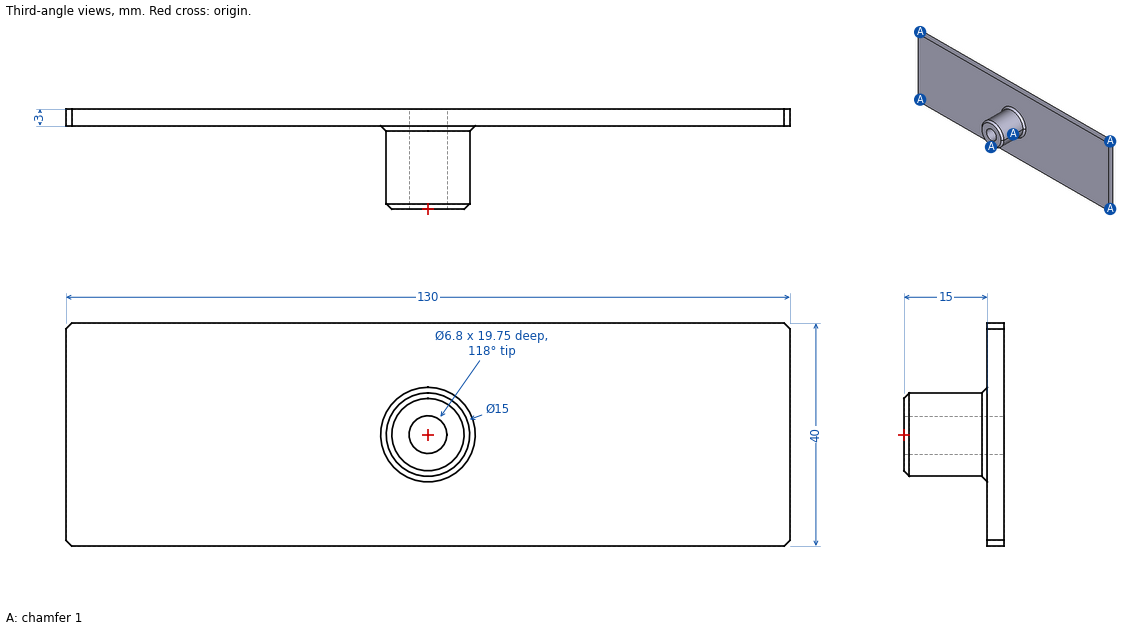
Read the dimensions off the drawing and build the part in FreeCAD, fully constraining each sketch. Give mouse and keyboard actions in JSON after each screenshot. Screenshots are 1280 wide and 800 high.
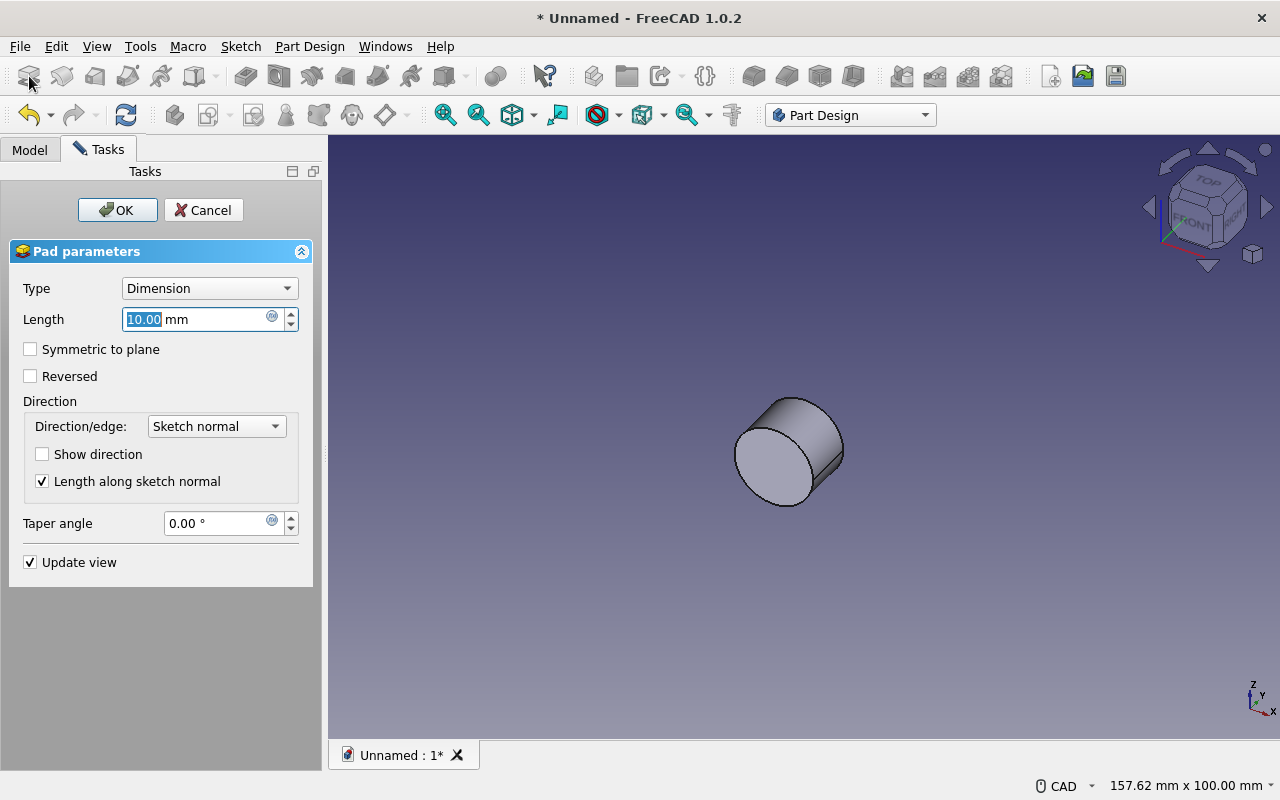
{"action": "type", "text": "15"}
{"action": "key", "text": "Tab"}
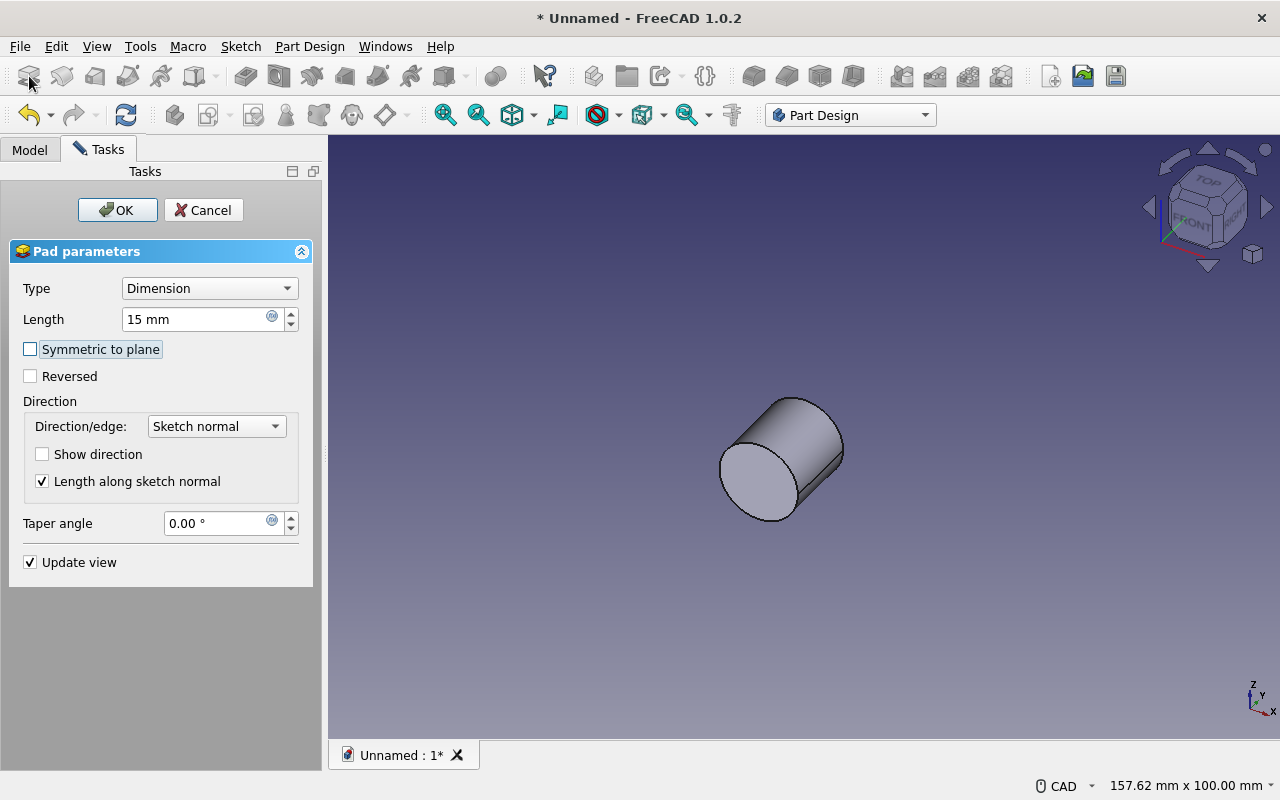
{"action": "left_click", "coordinate": [31, 376]}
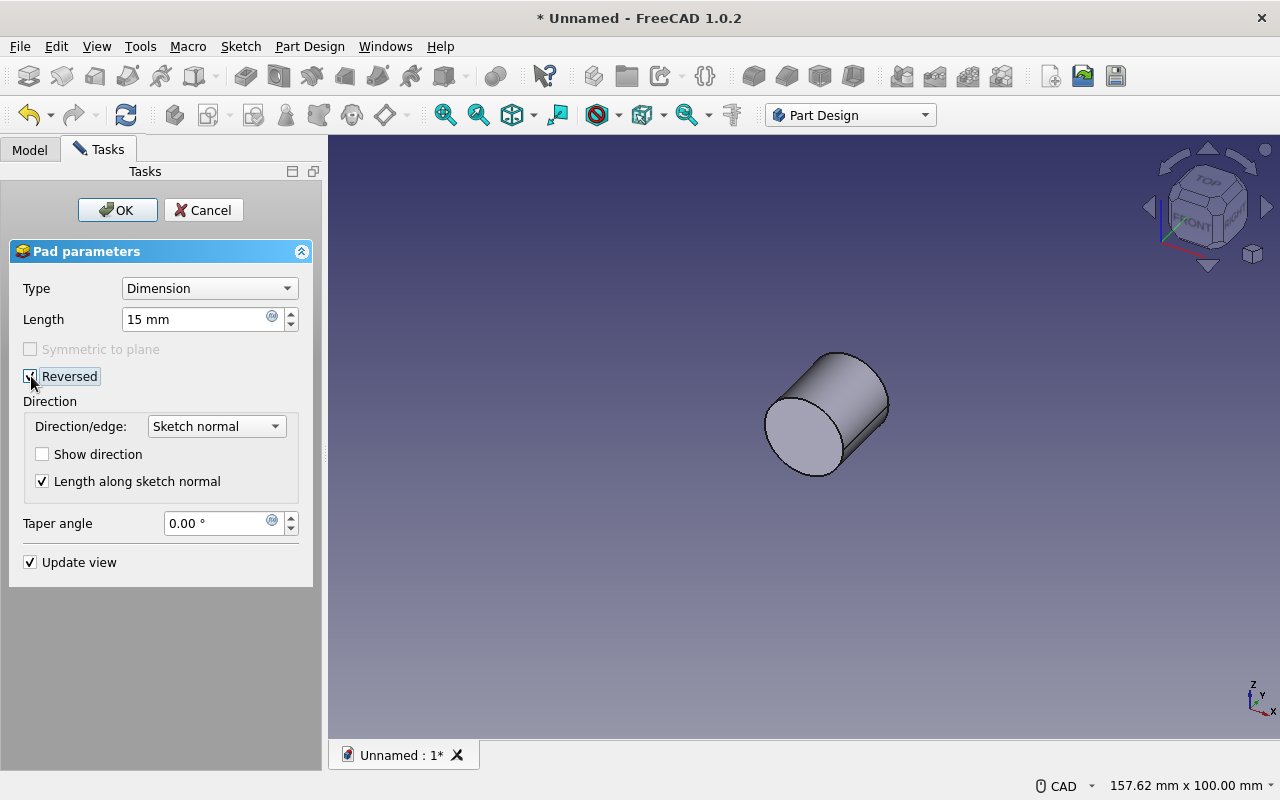
{"action": "left_click", "coordinate": [118, 210]}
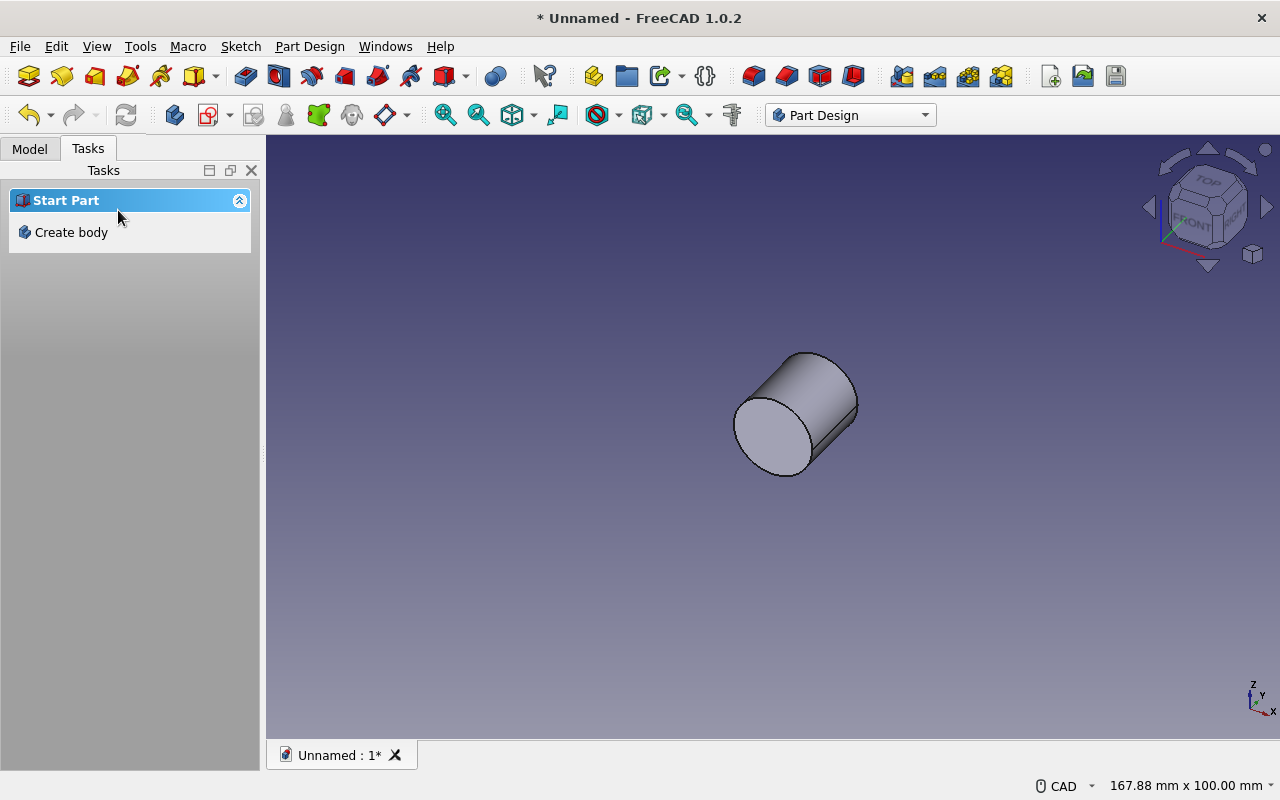
{"action": "left_click", "coordinate": [446, 116]}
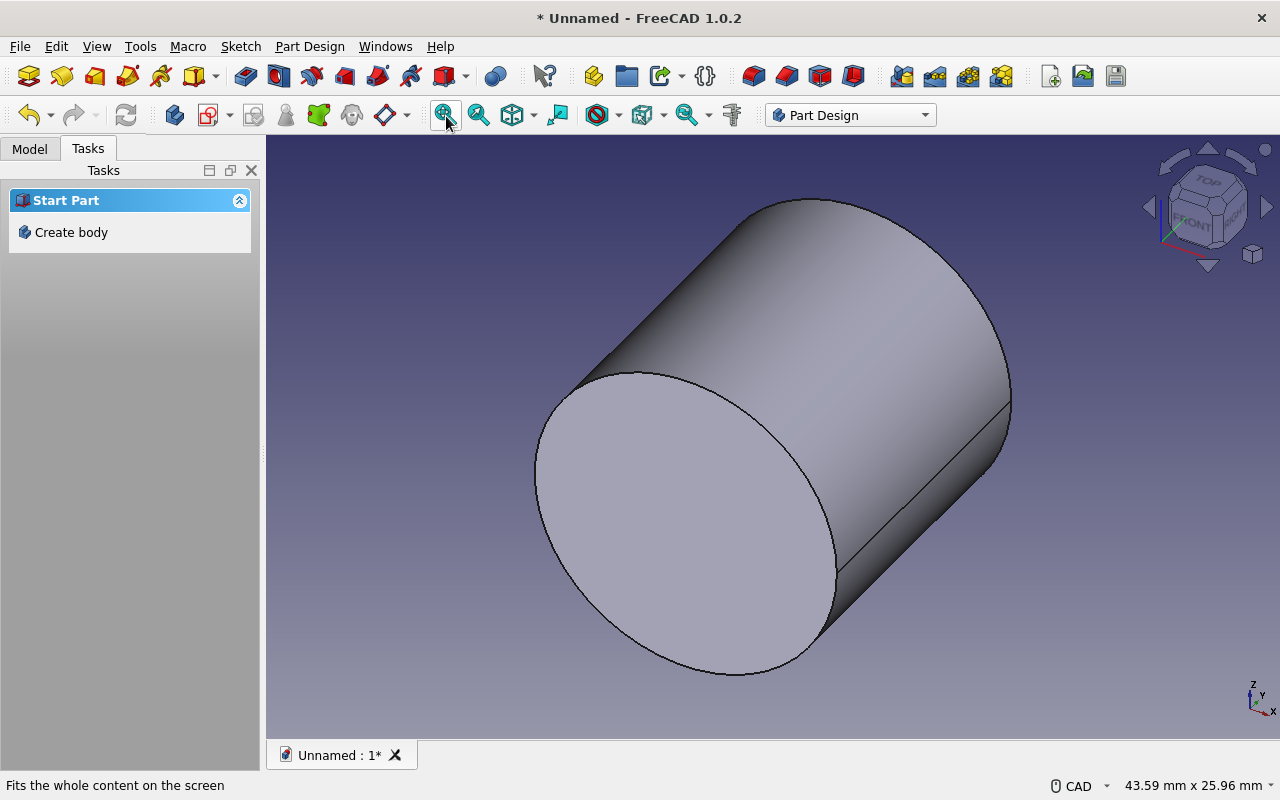
{"action": "key", "text": "4"}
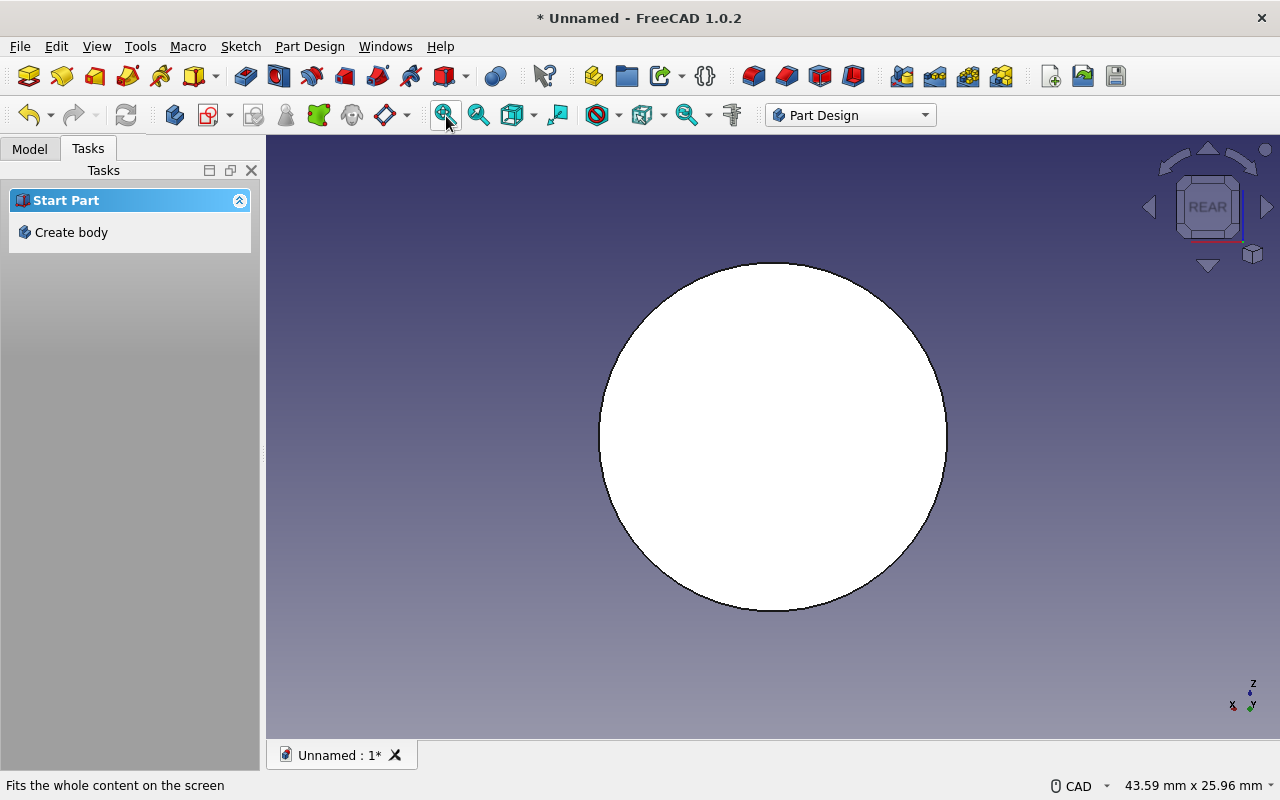
{"action": "left_click", "coordinate": [773, 436]}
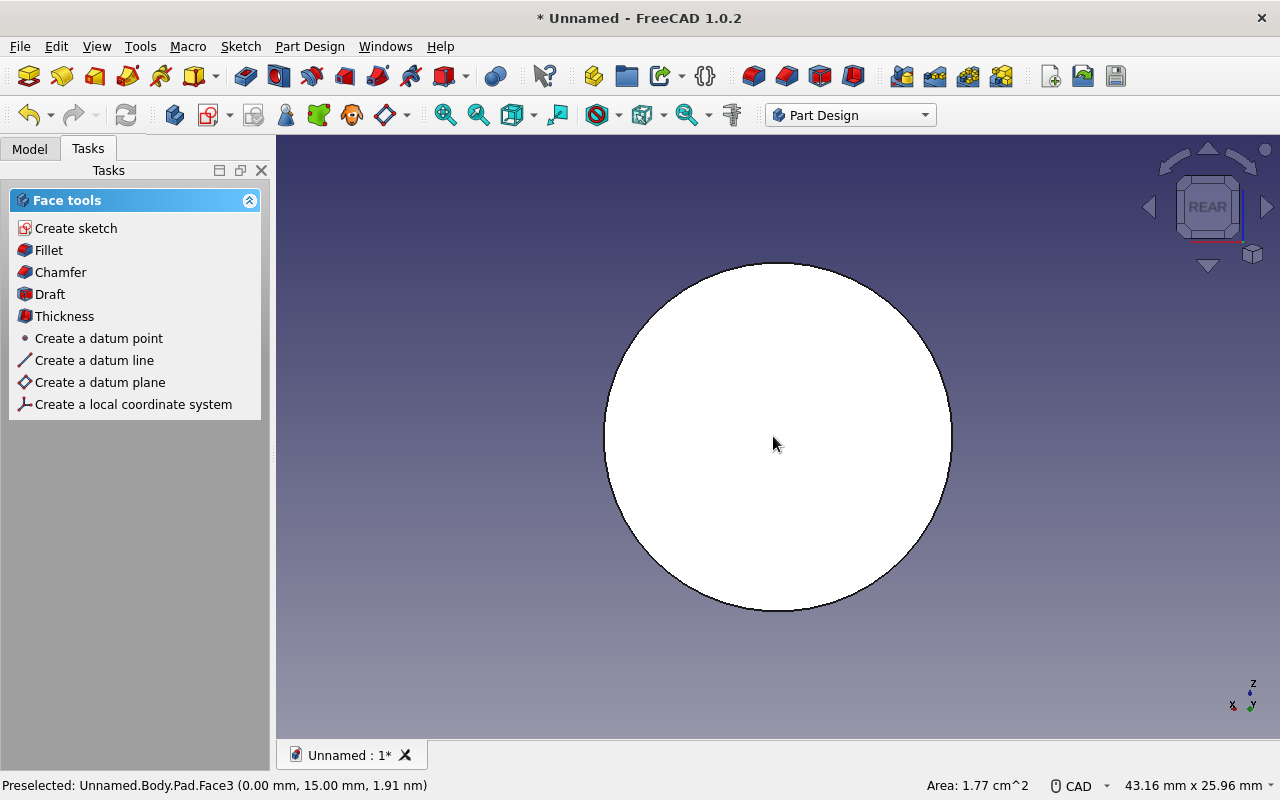
{"action": "left_click", "coordinate": [208, 116]}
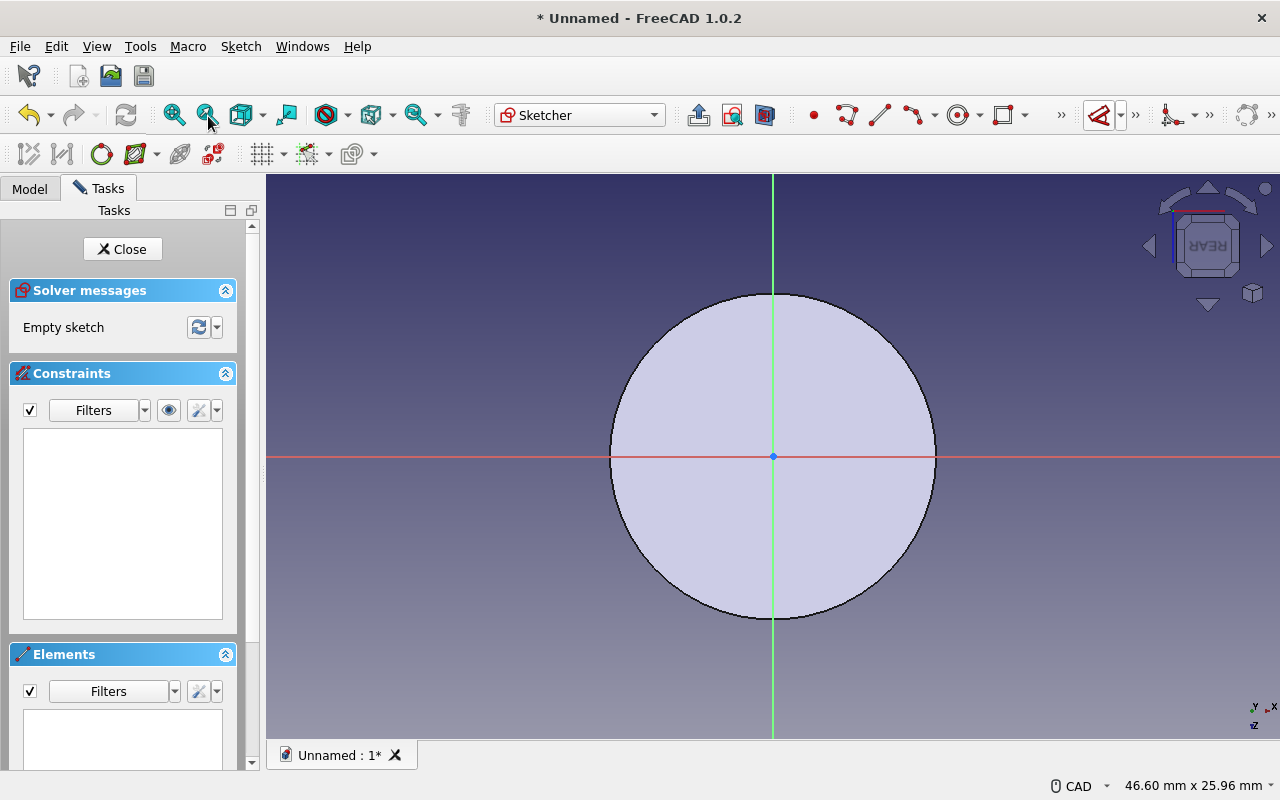
{"action": "scroll", "coordinate": [687, 457], "scroll_direction": "down", "scroll_amount": 8}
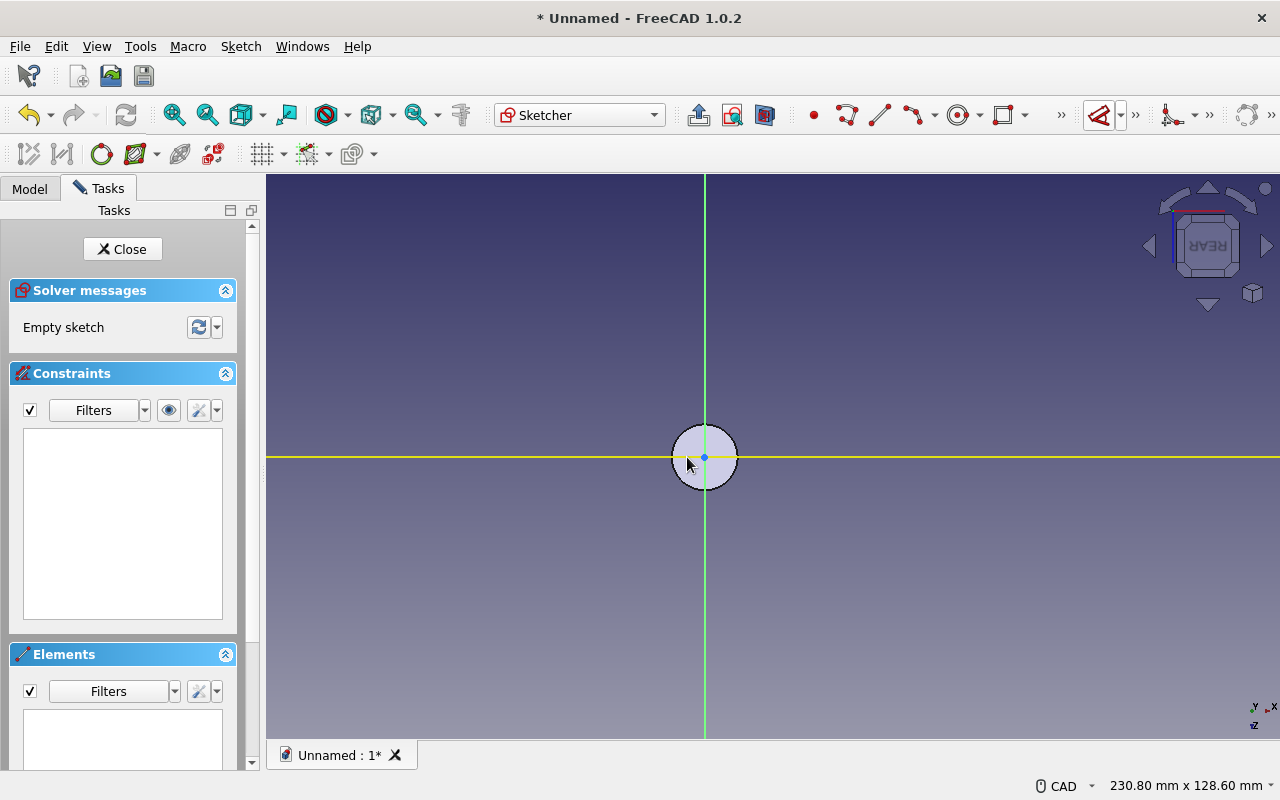
{"action": "left_click", "coordinate": [1024, 116]}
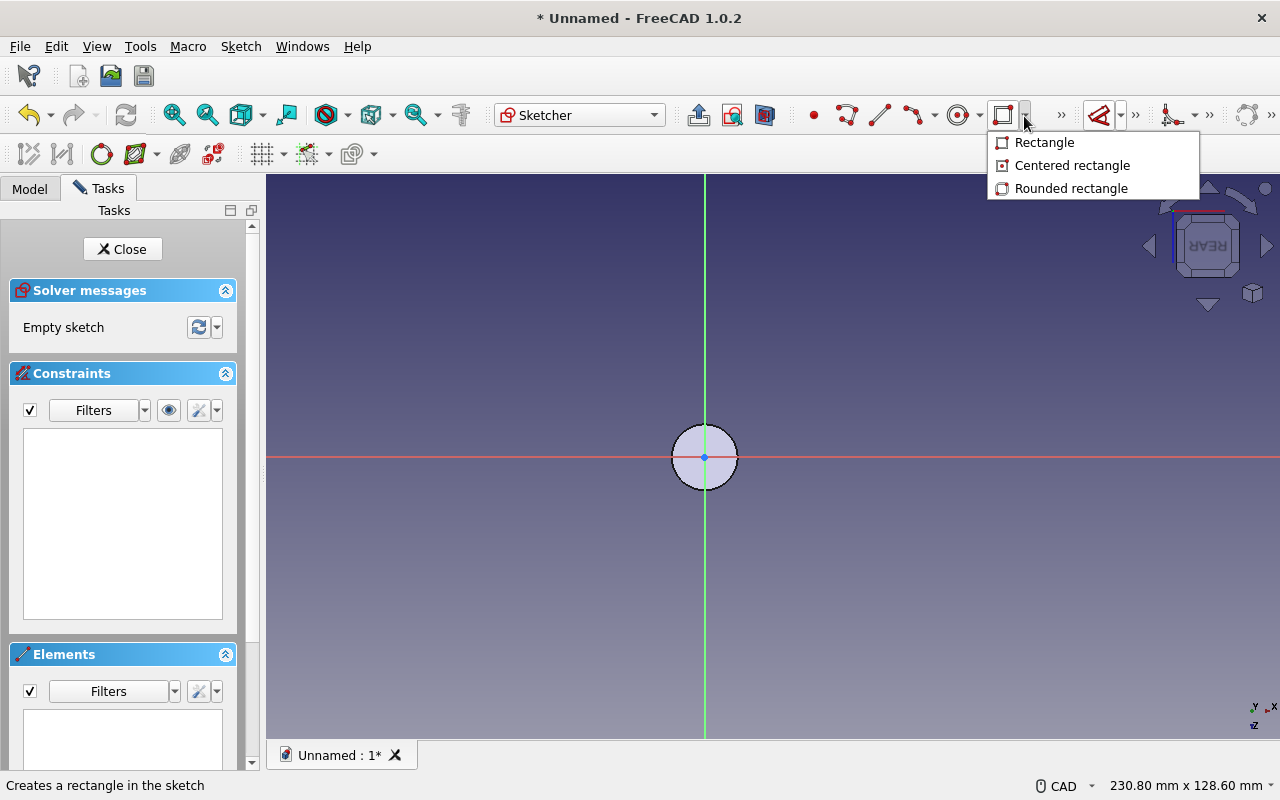
{"action": "left_click", "coordinate": [1094, 166]}